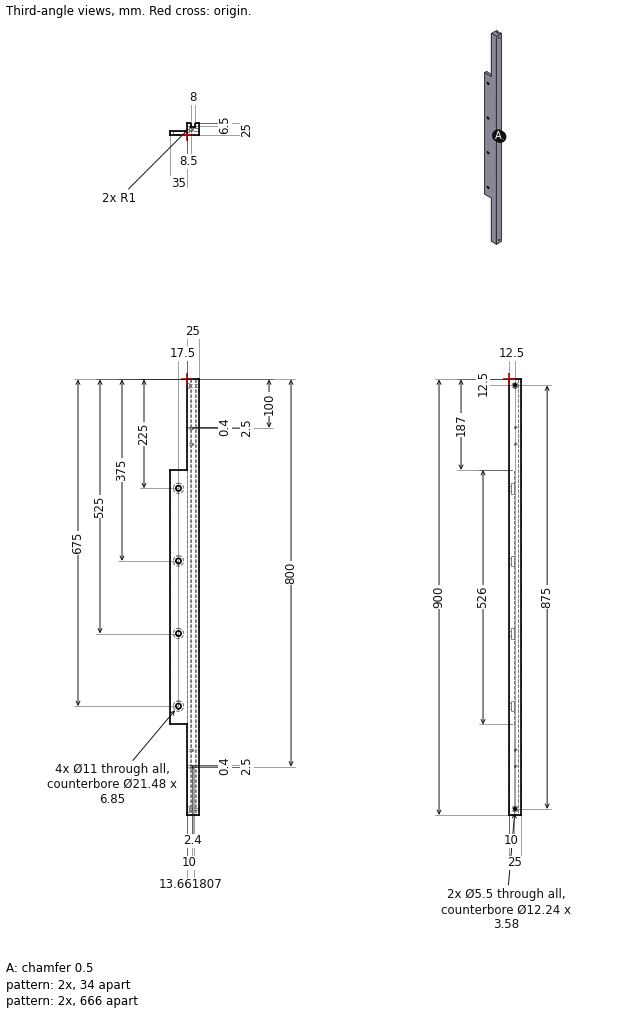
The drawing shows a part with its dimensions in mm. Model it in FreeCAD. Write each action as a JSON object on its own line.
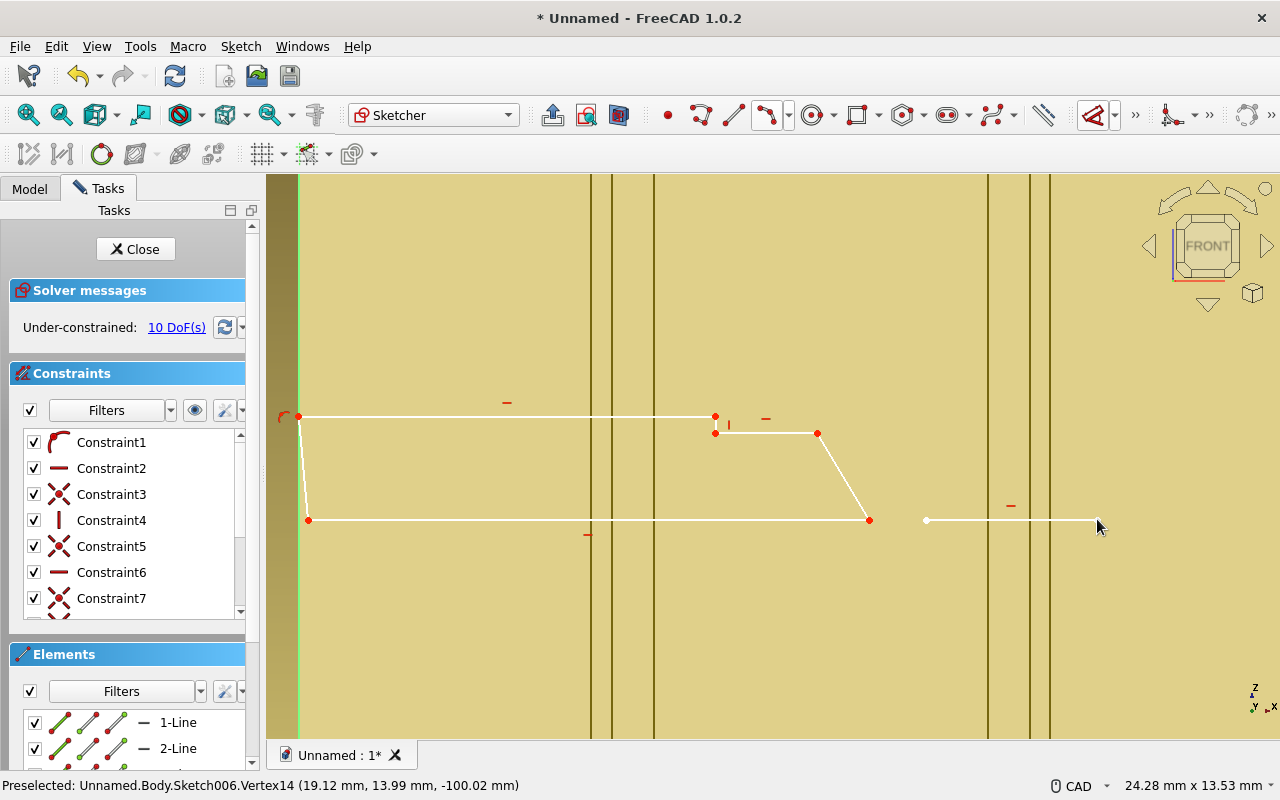
{"action": "left_click", "coordinate": [977, 520]}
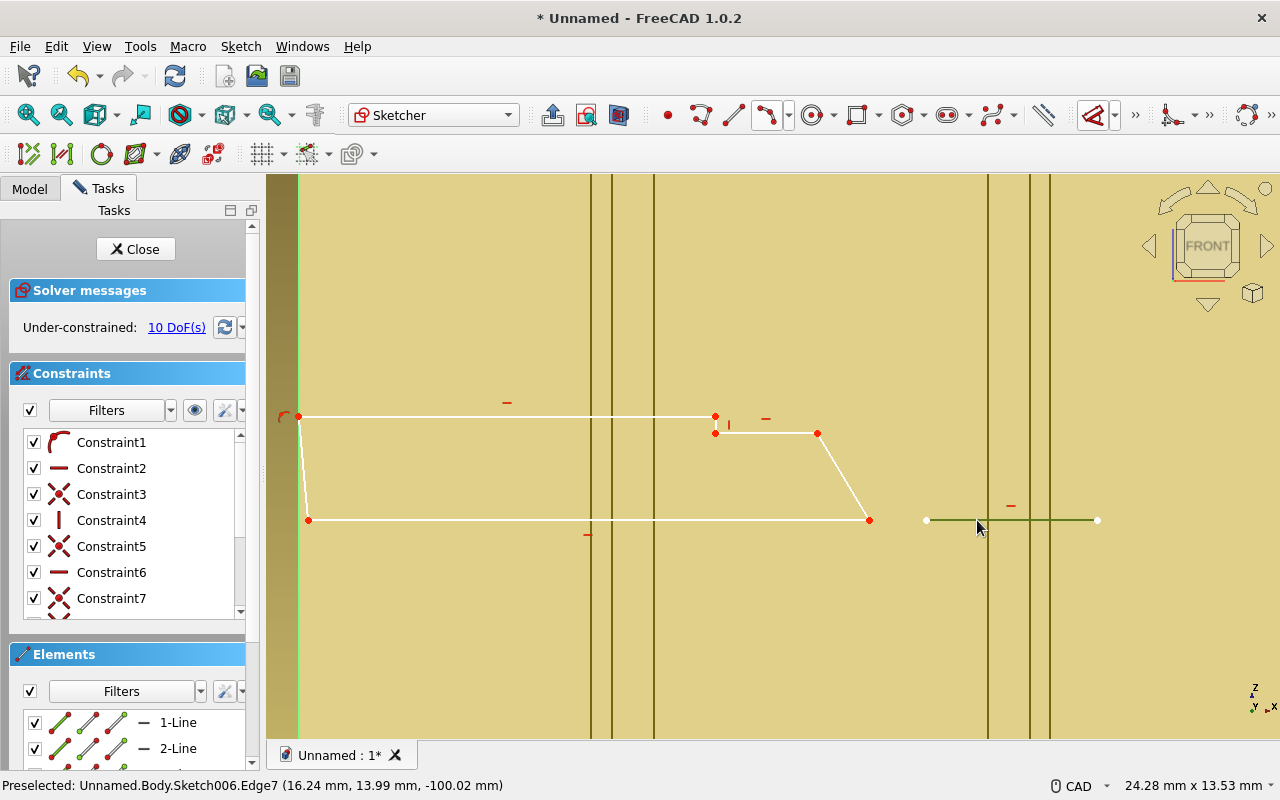
{"action": "key", "text": "g n"}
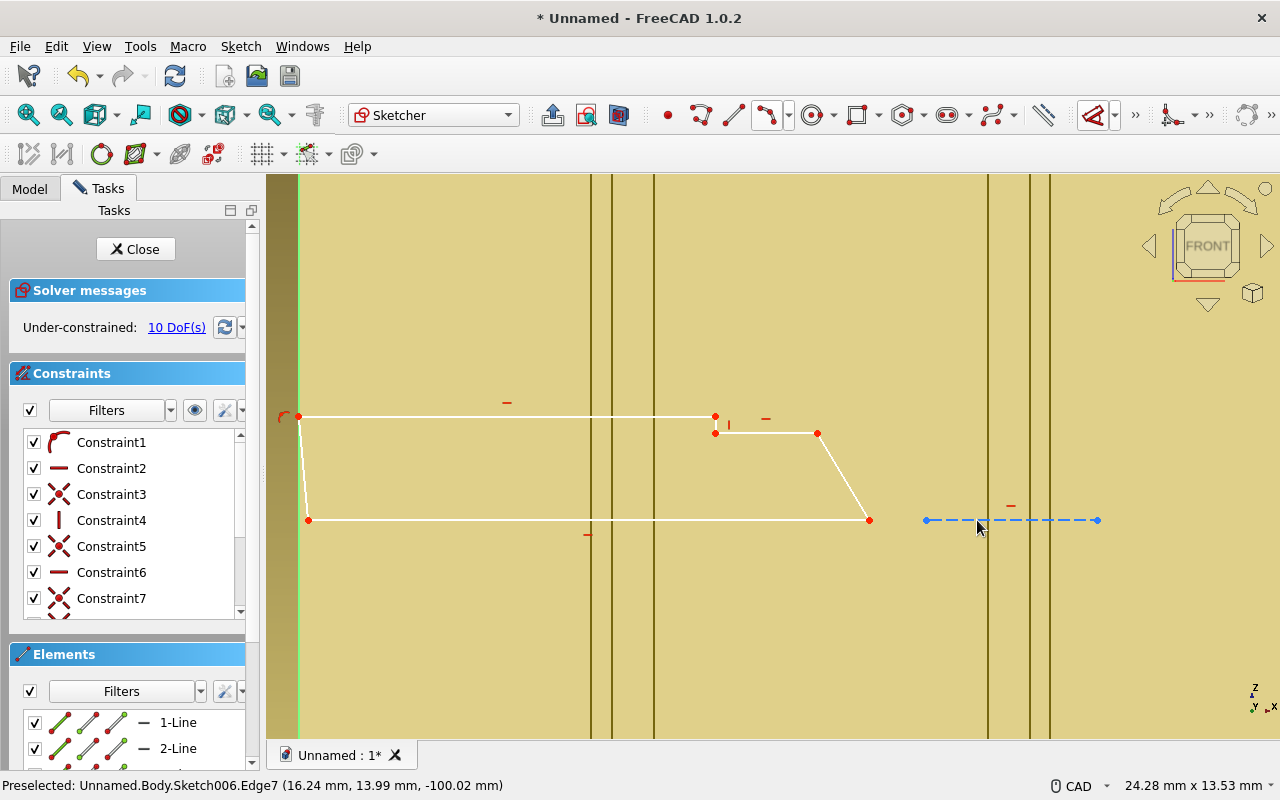
{"action": "left_click", "coordinate": [302, 448]}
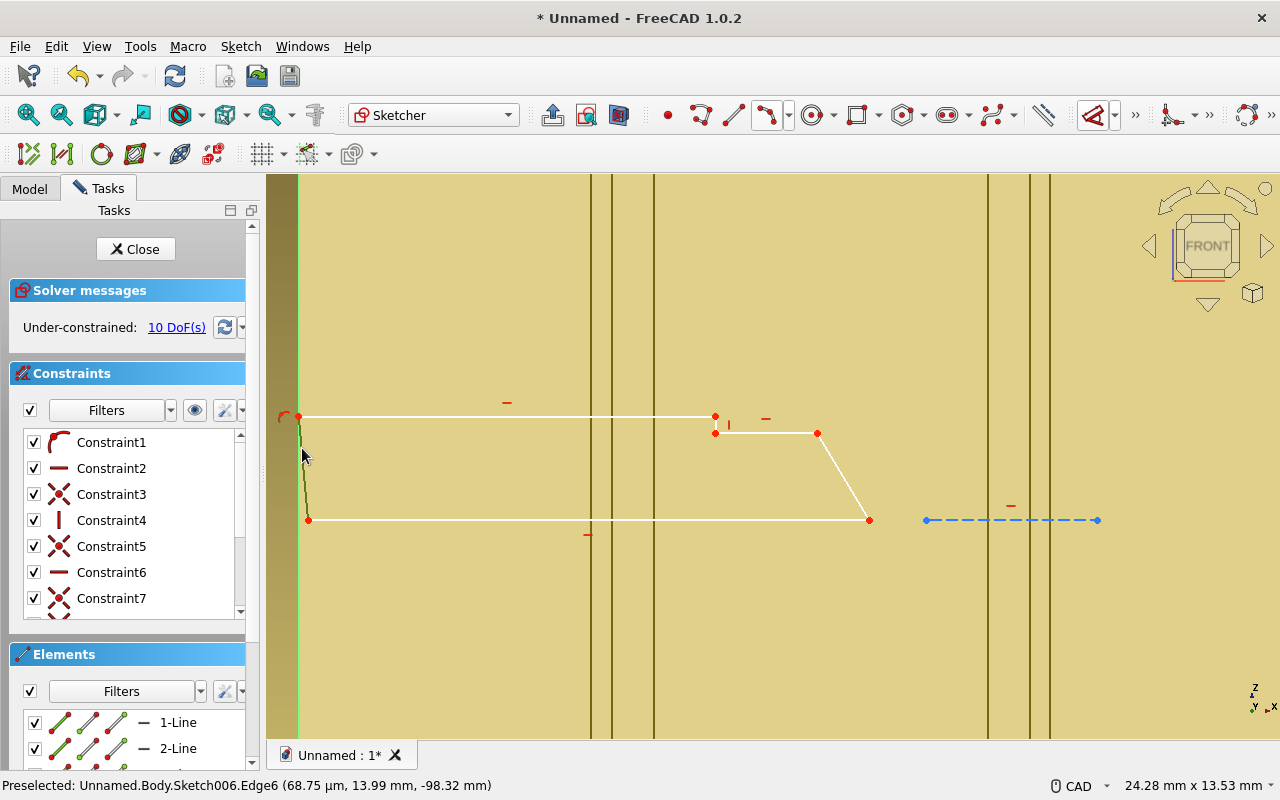
{"action": "key", "text": "v"}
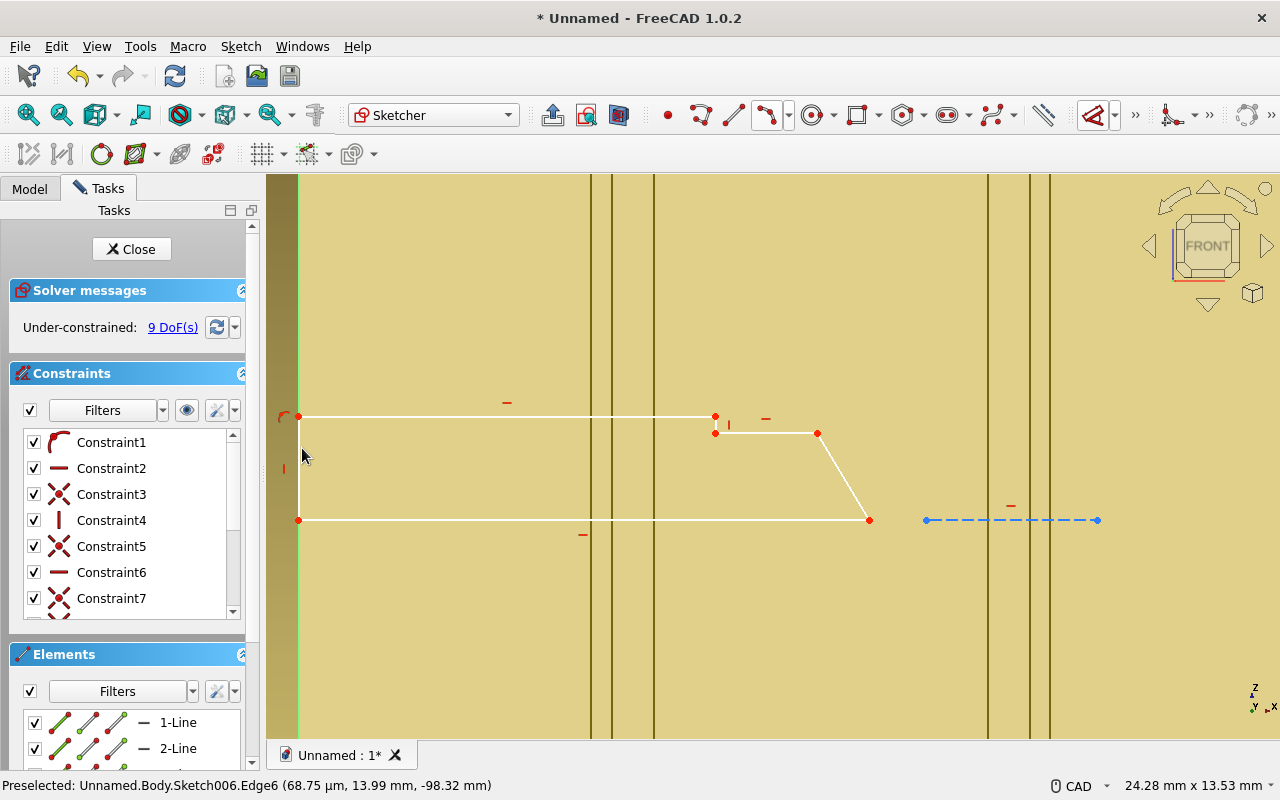
{"action": "left_click", "coordinate": [424, 417]}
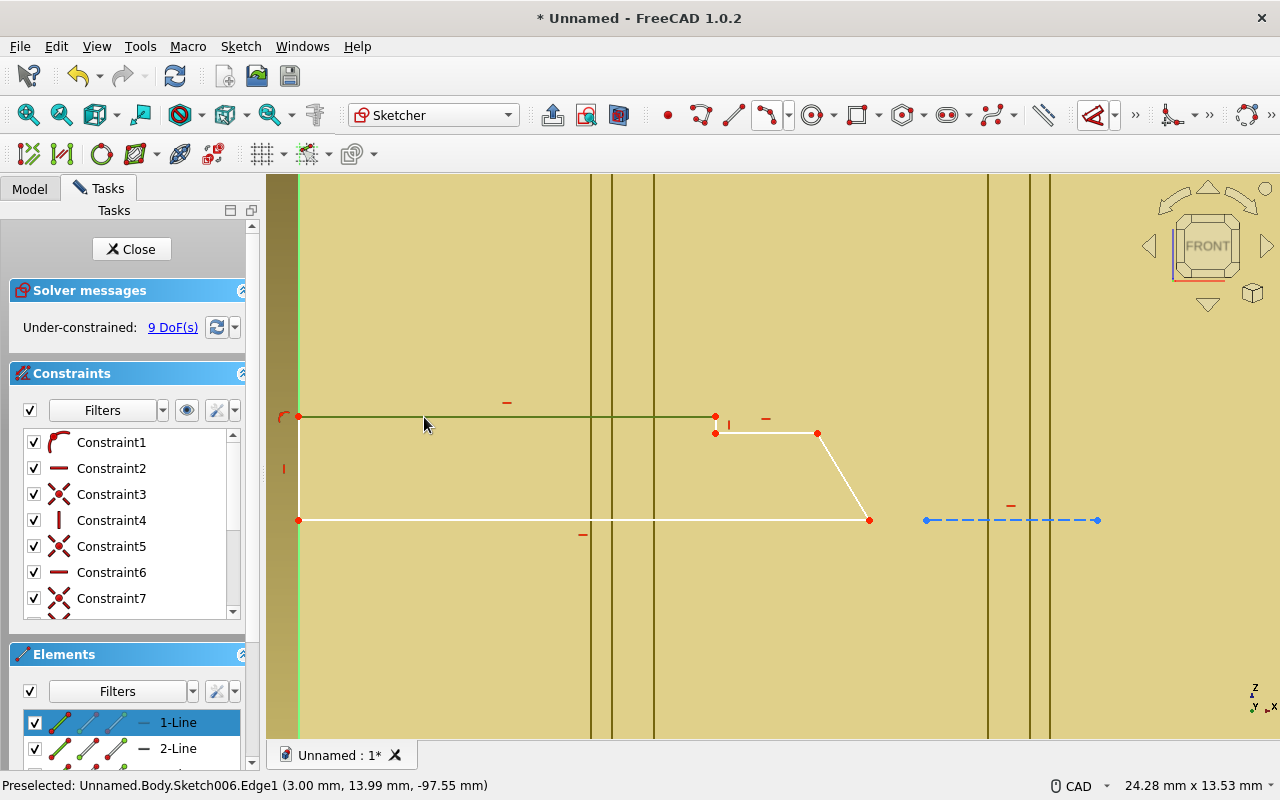
{"action": "left_click", "coordinate": [1114, 116]}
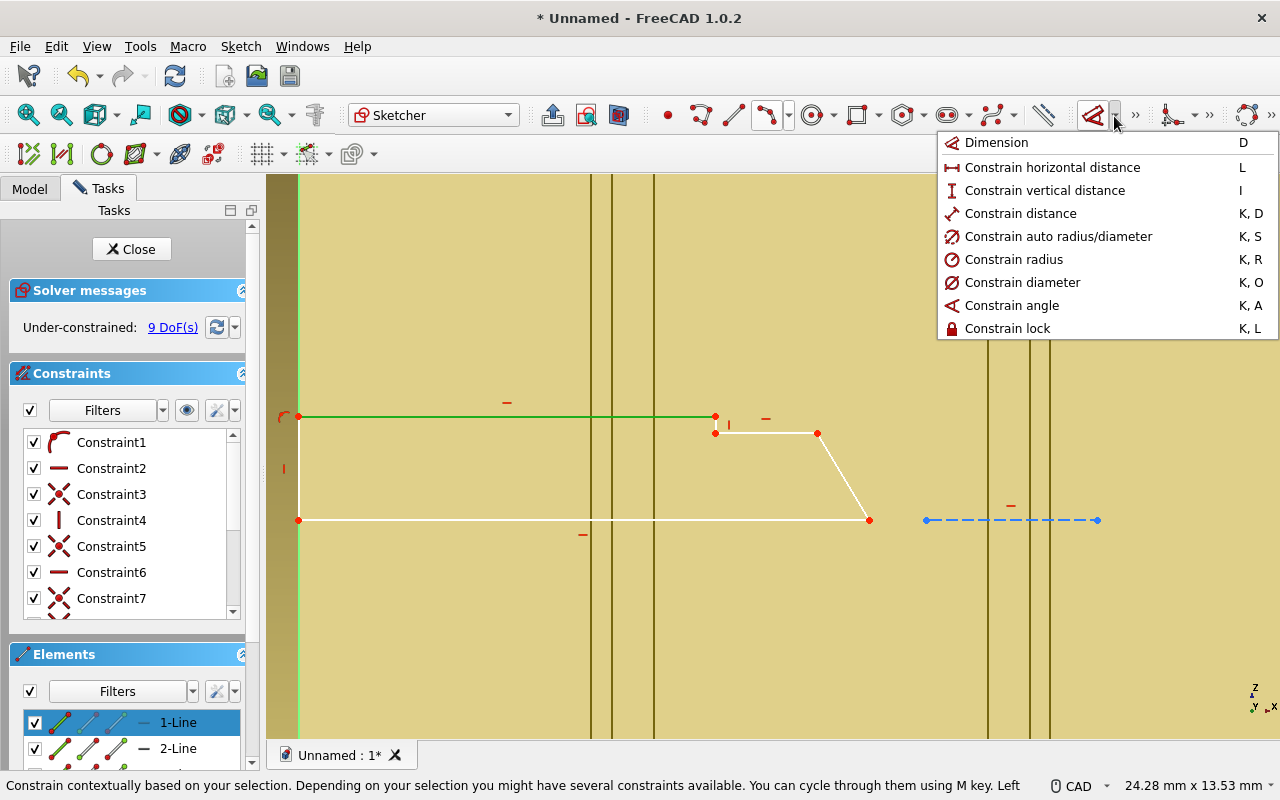
{"action": "left_click", "coordinate": [1108, 168]}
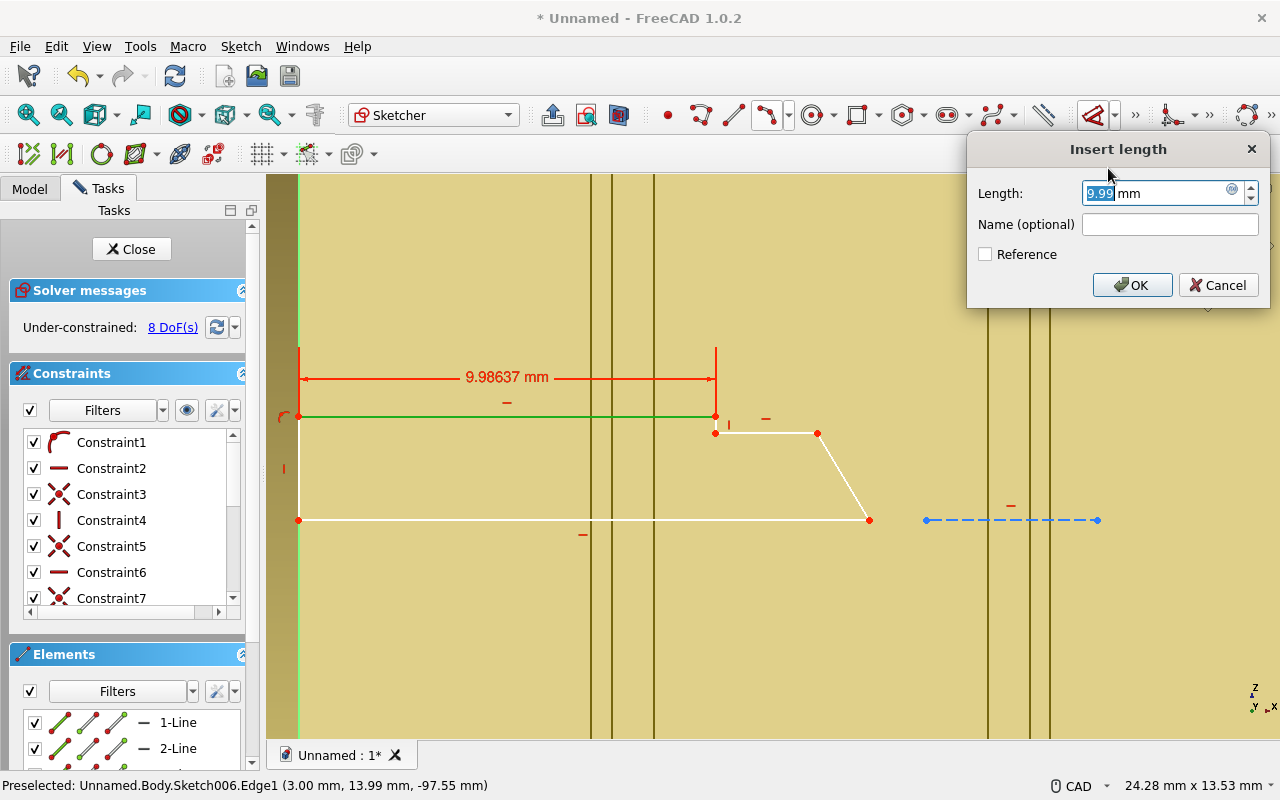
{"action": "type", "text": "10"}
{"action": "key", "text": "Return"}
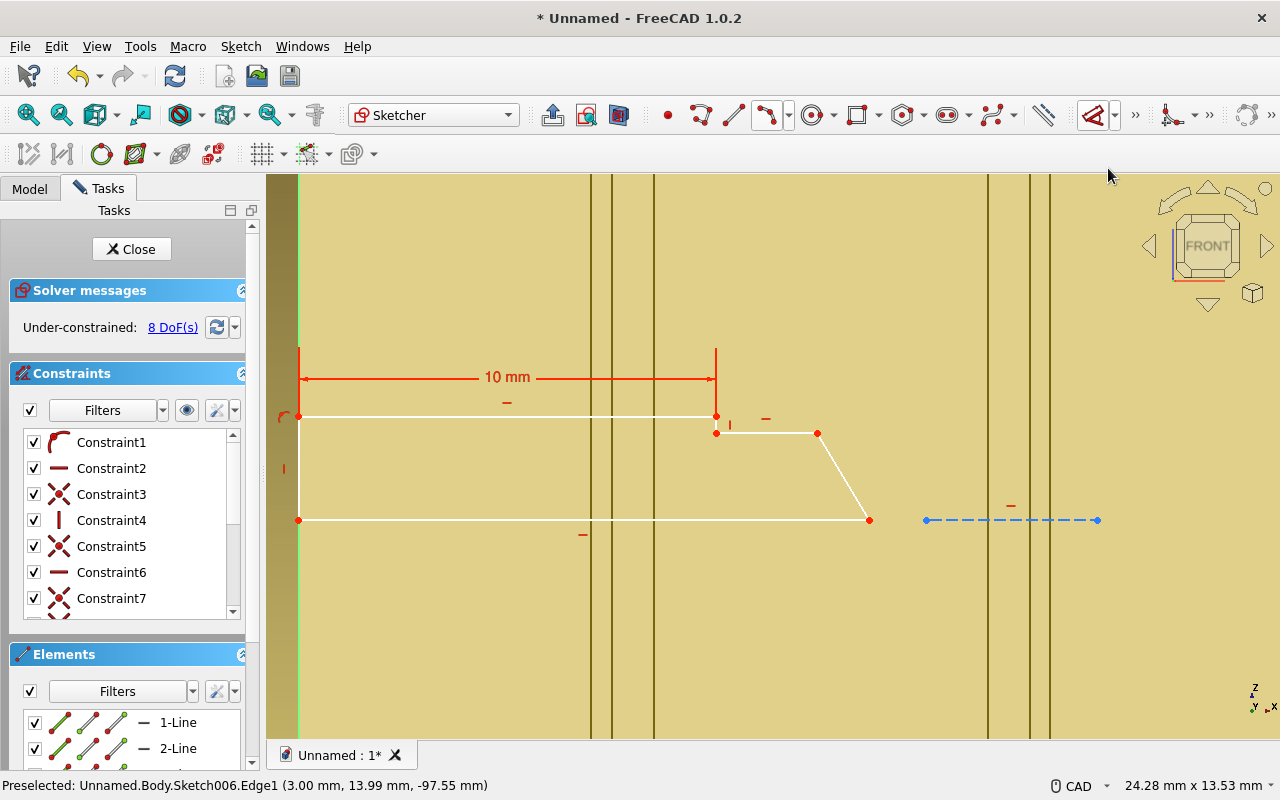
{"action": "scroll", "coordinate": [716, 425], "scroll_direction": "up", "scroll_amount": 5}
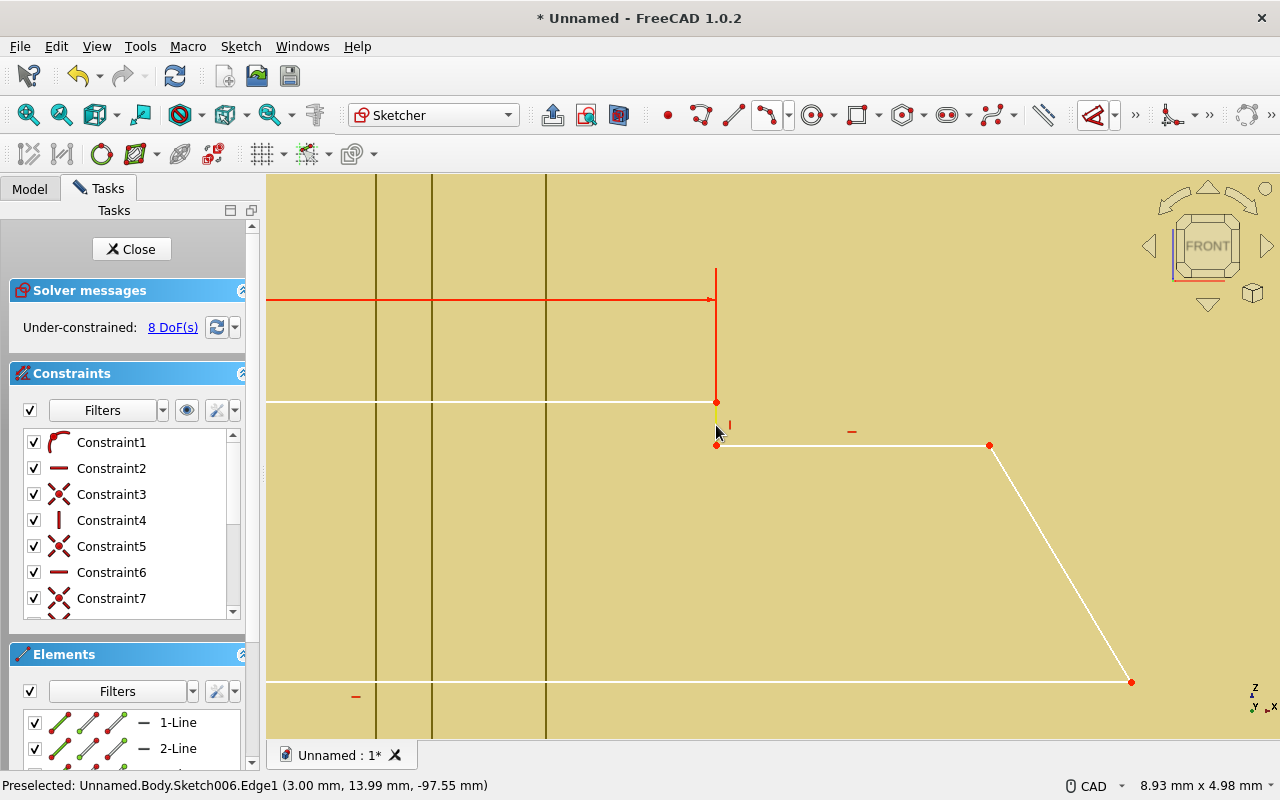
{"action": "left_click", "coordinate": [716, 424]}